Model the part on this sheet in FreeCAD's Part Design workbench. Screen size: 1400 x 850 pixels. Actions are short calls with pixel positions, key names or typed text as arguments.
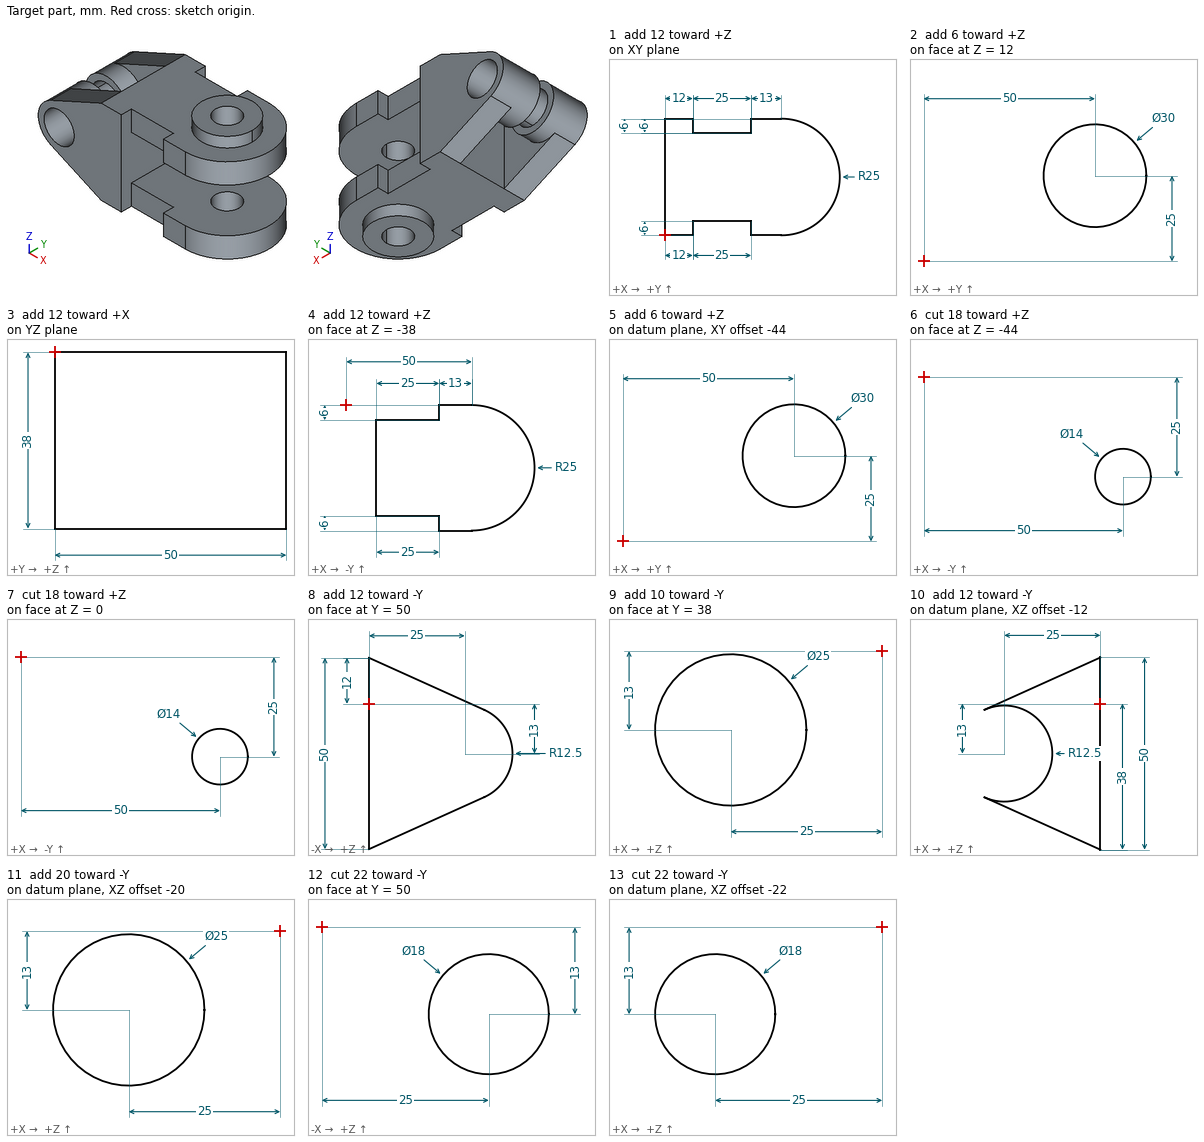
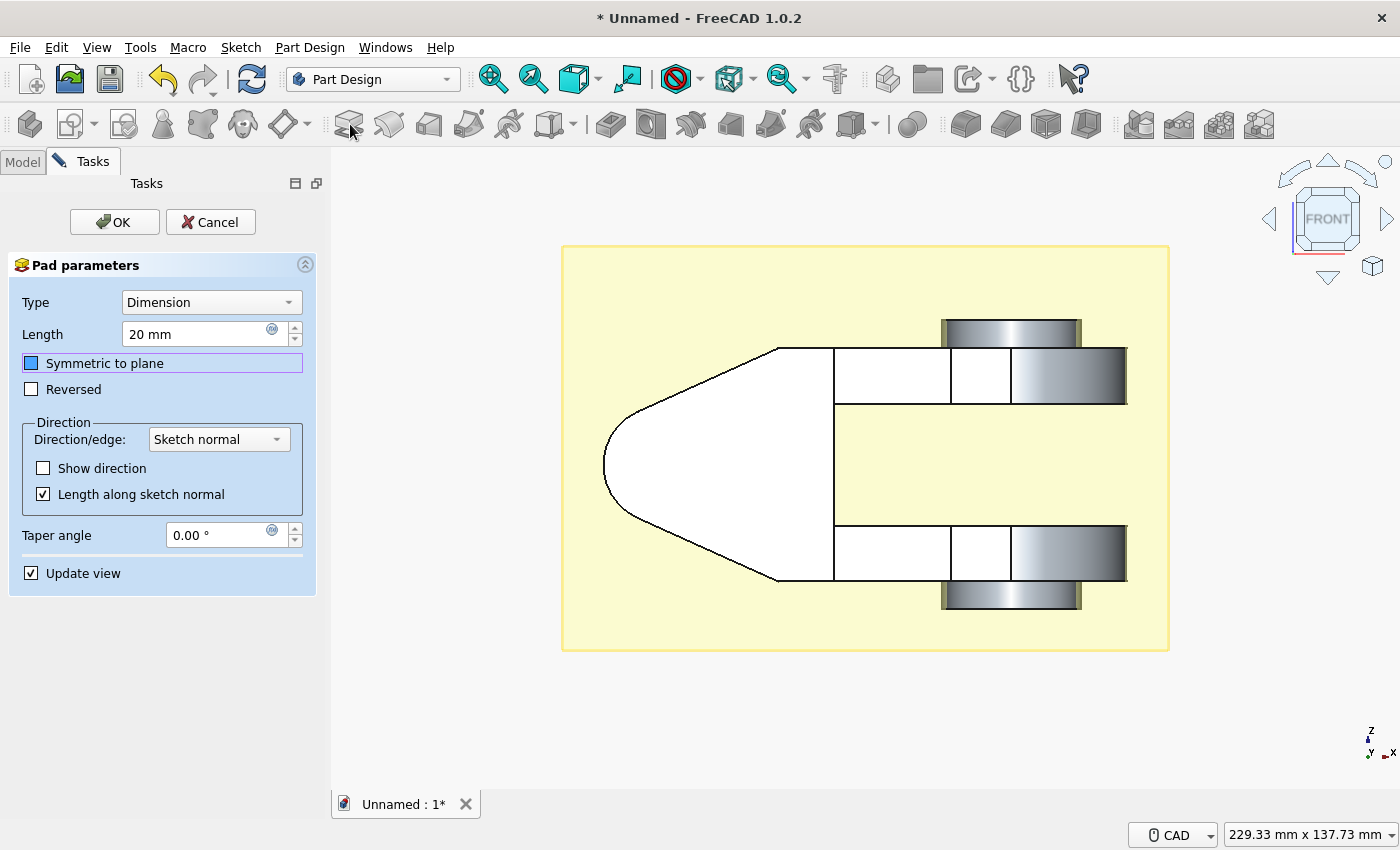
click(115, 222)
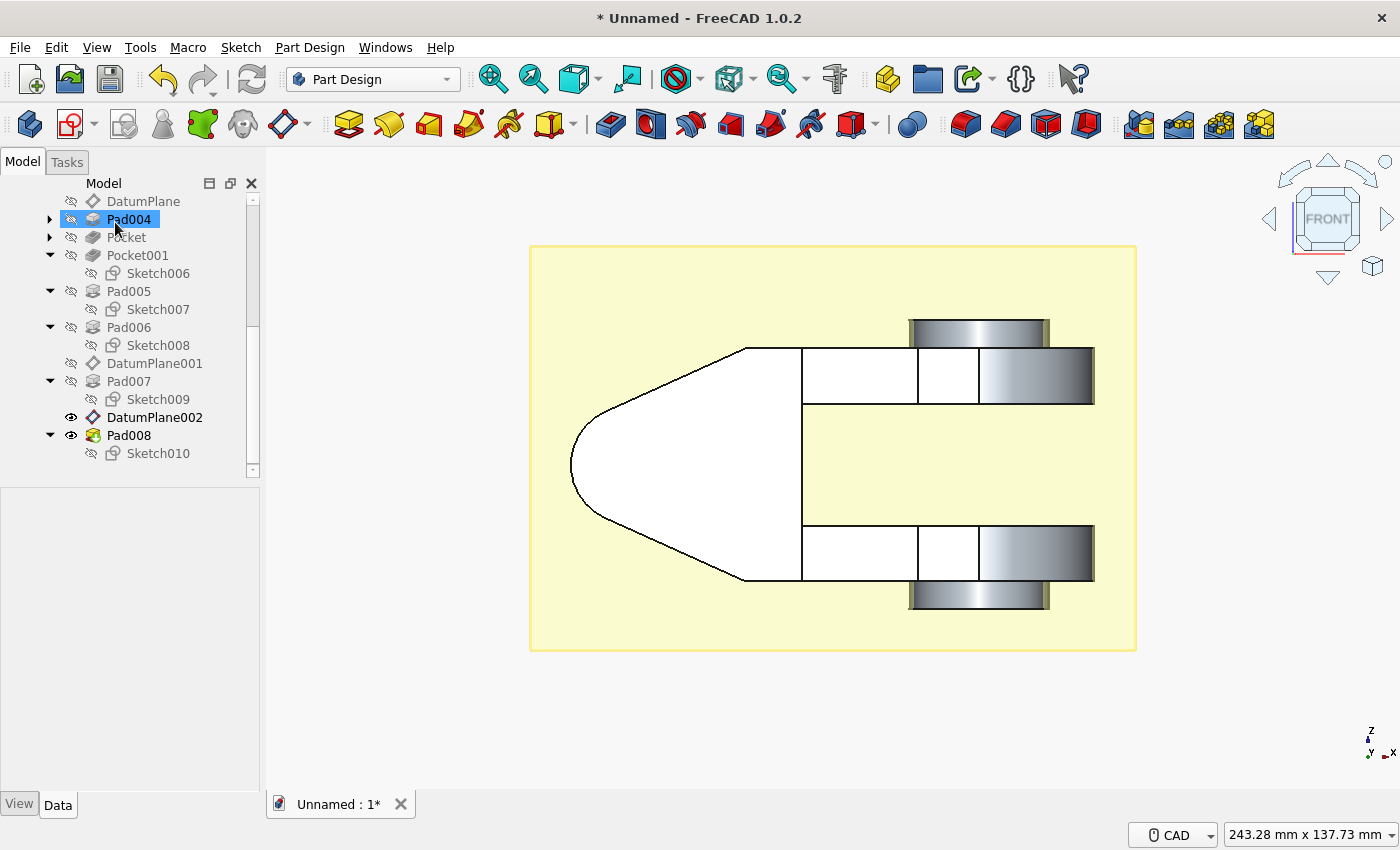
click(116, 417)
key(space)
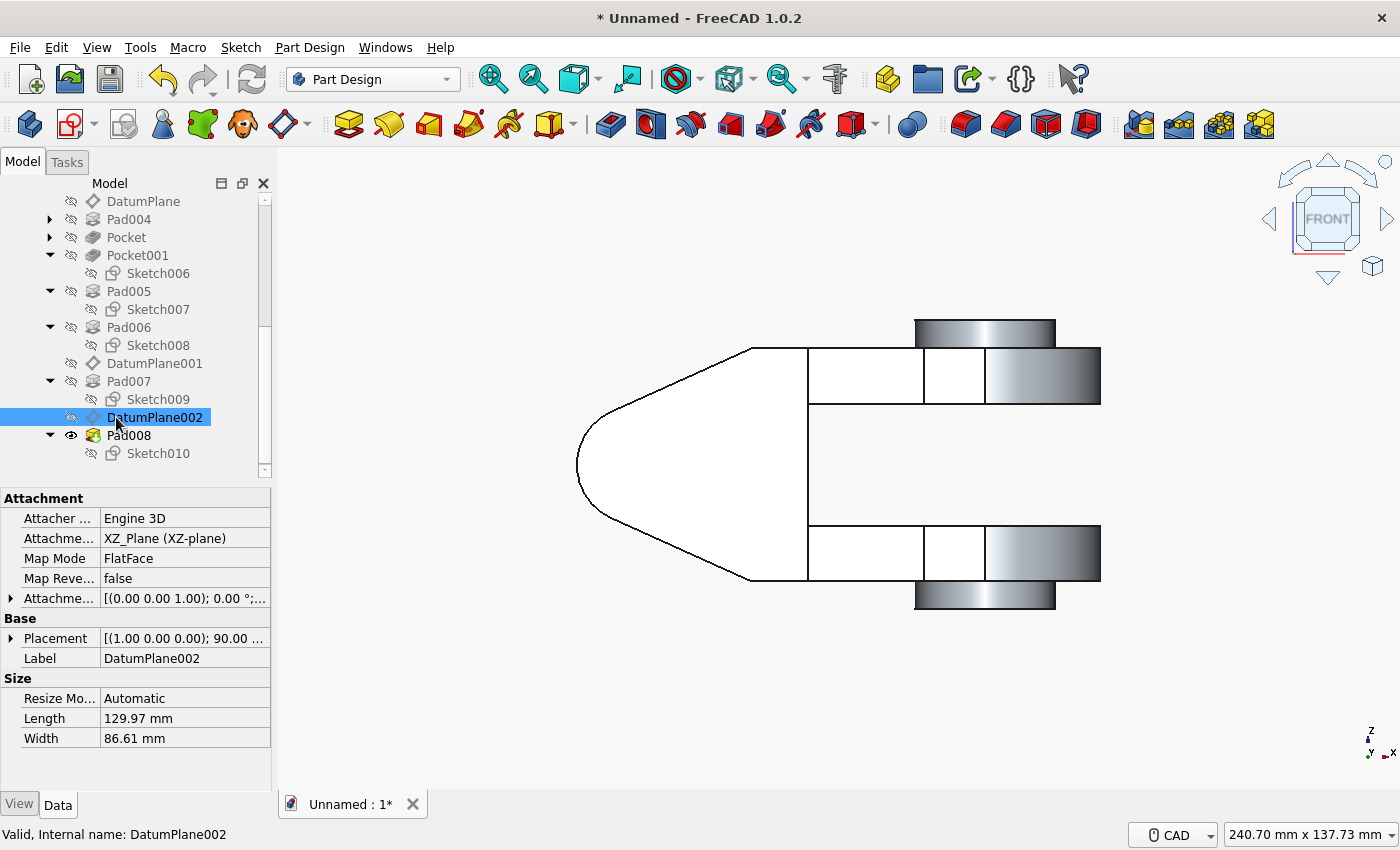
key(4)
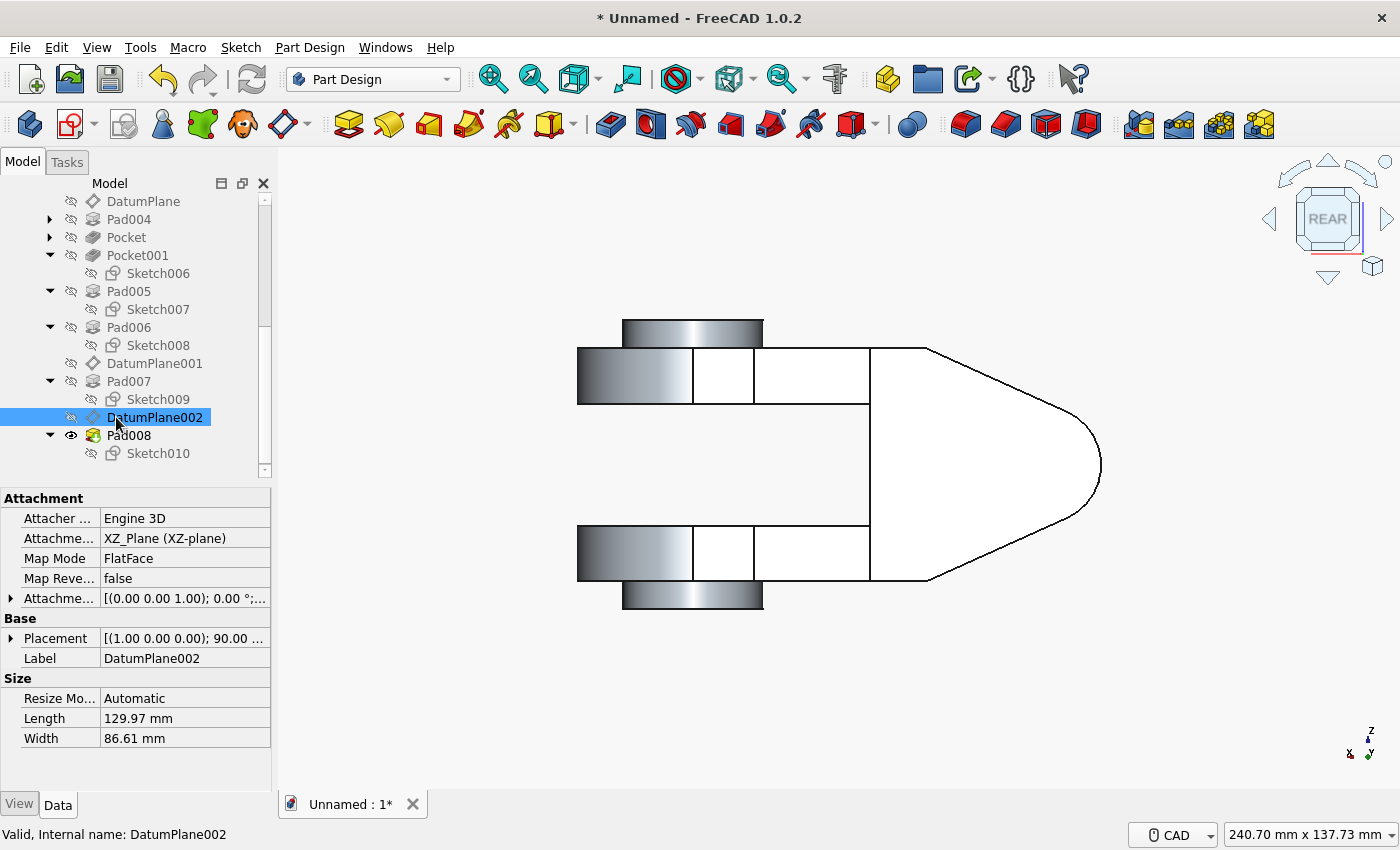
click(953, 464)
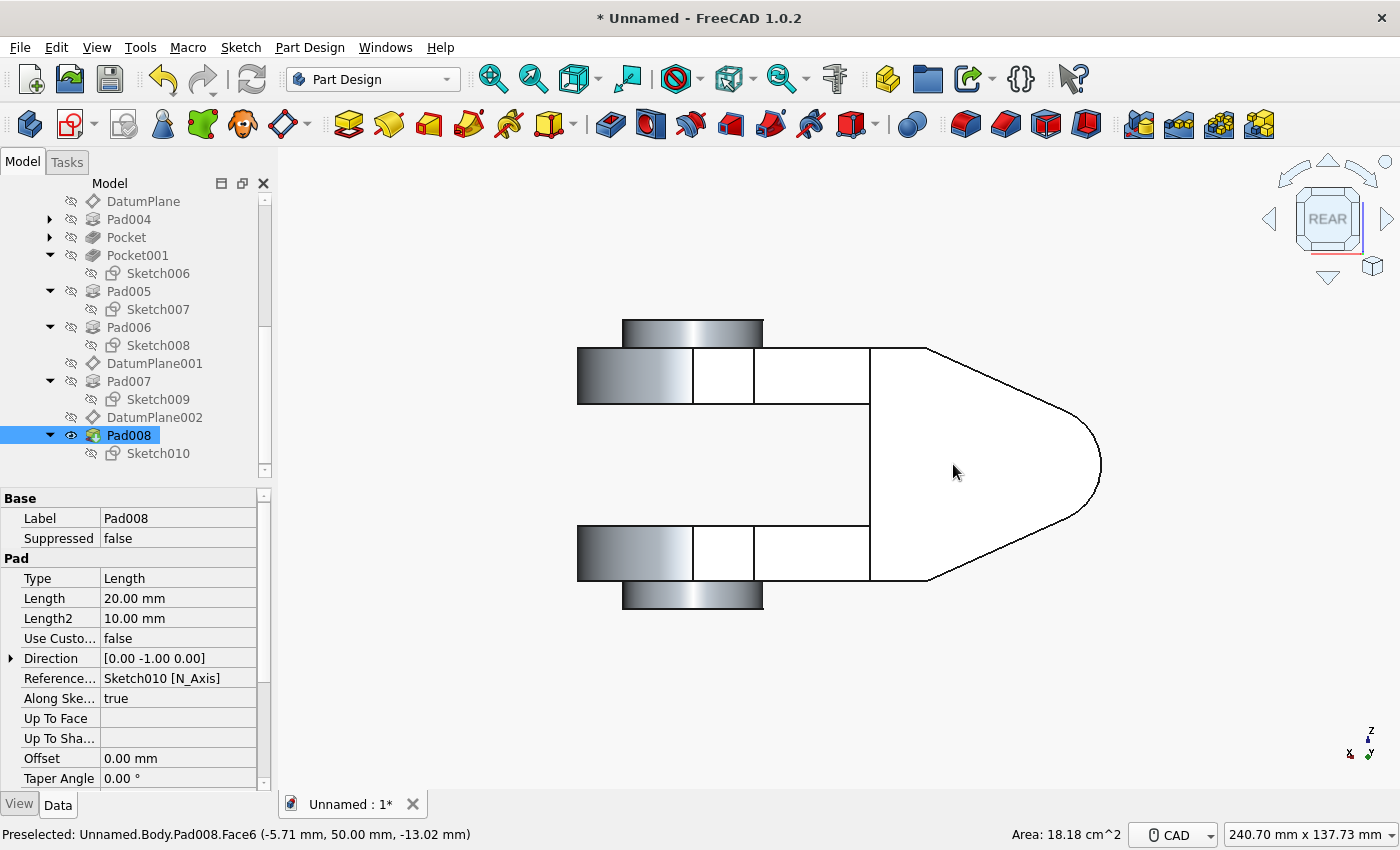
click(70, 124)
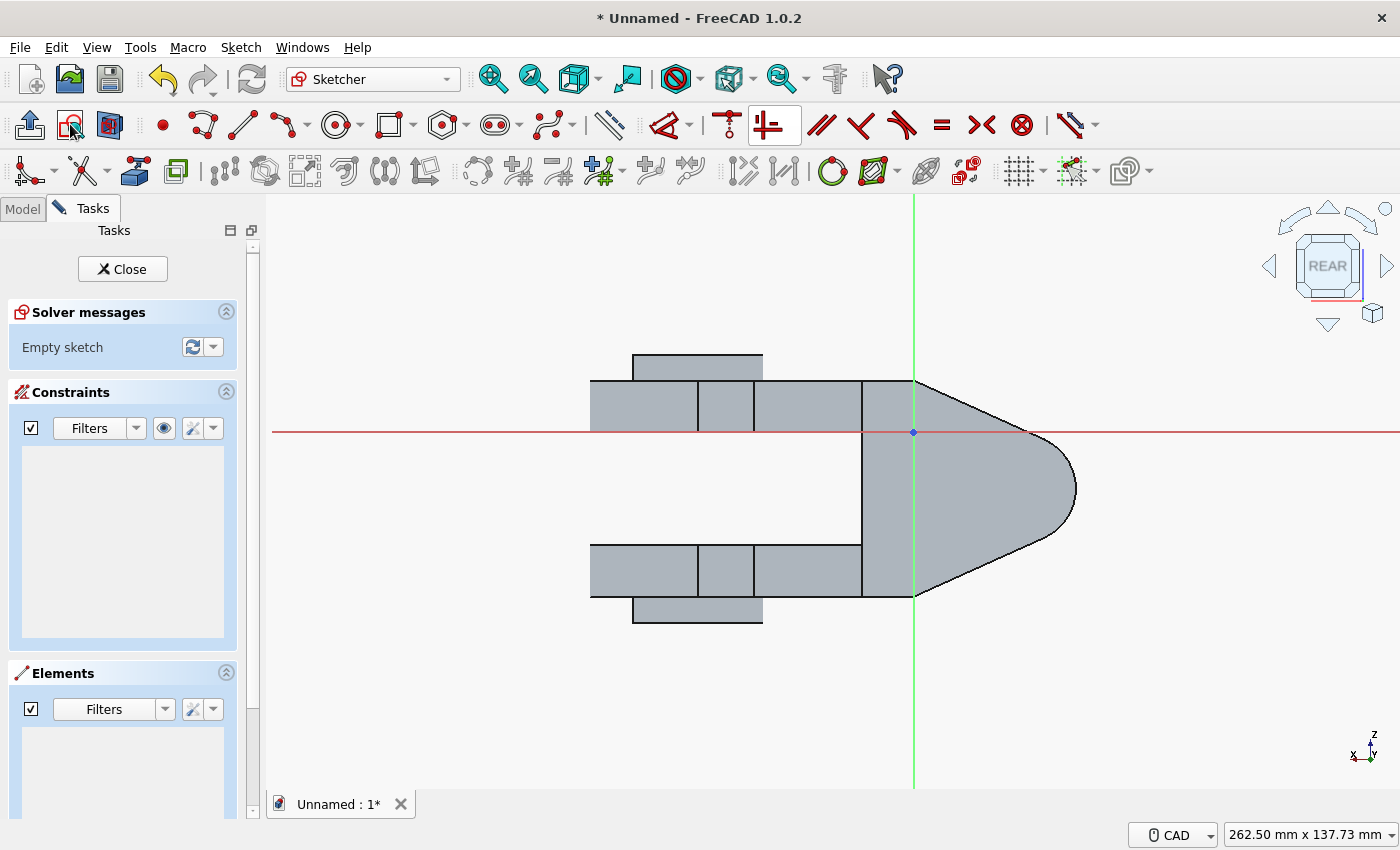
scroll(1060, 476, up, 7)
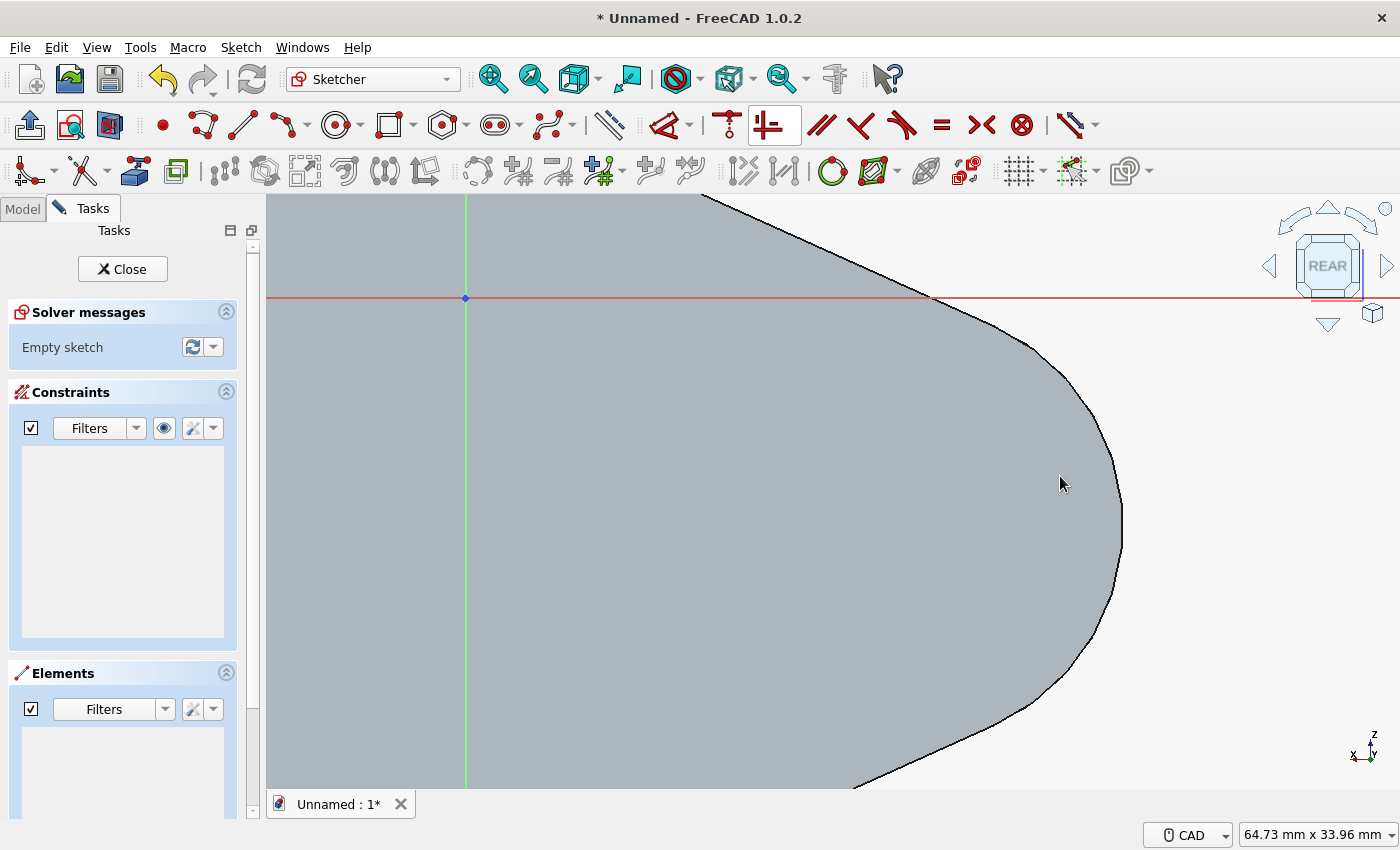
click(336, 126)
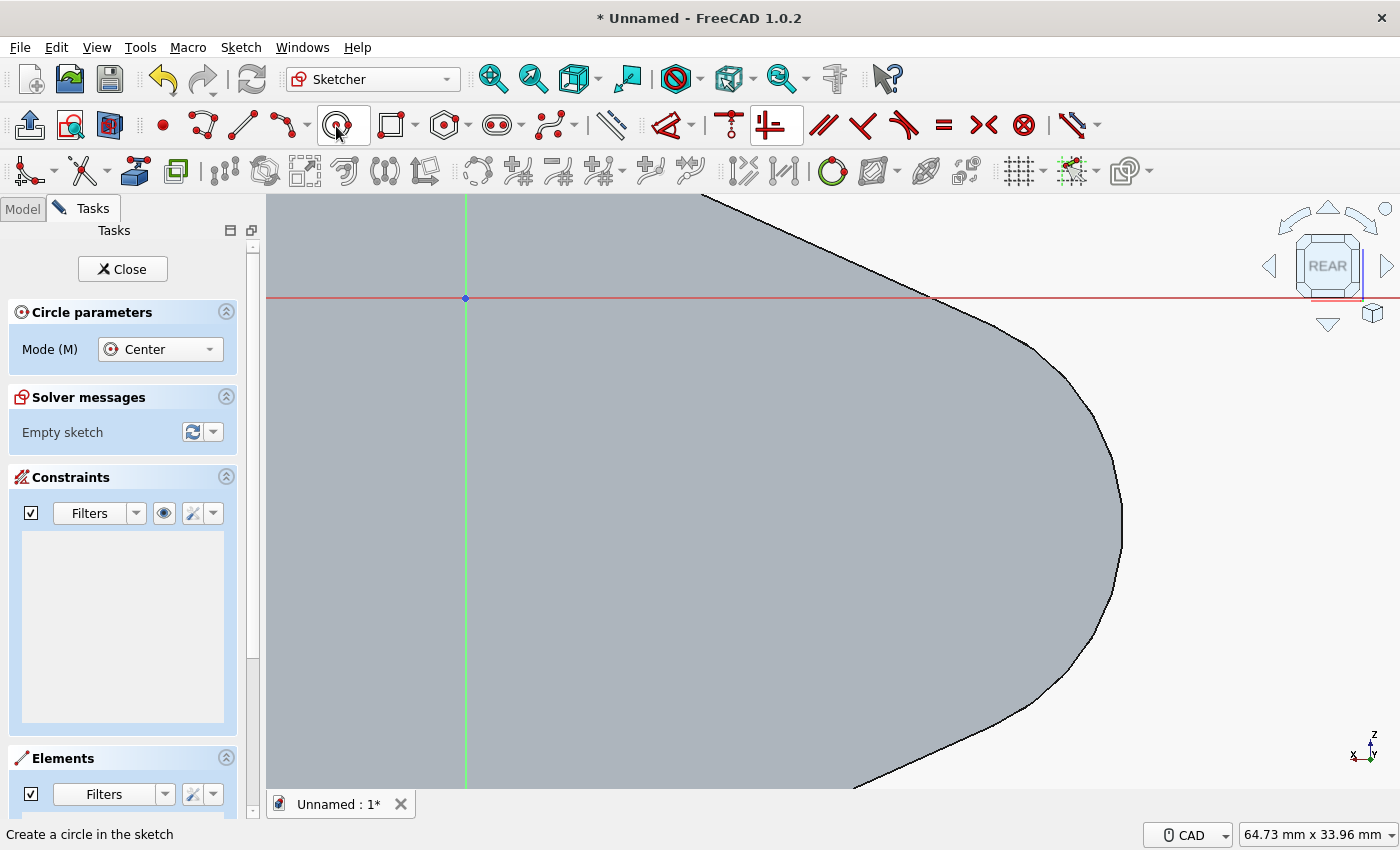
click(904, 526)
click(1015, 414)
key(Escape)